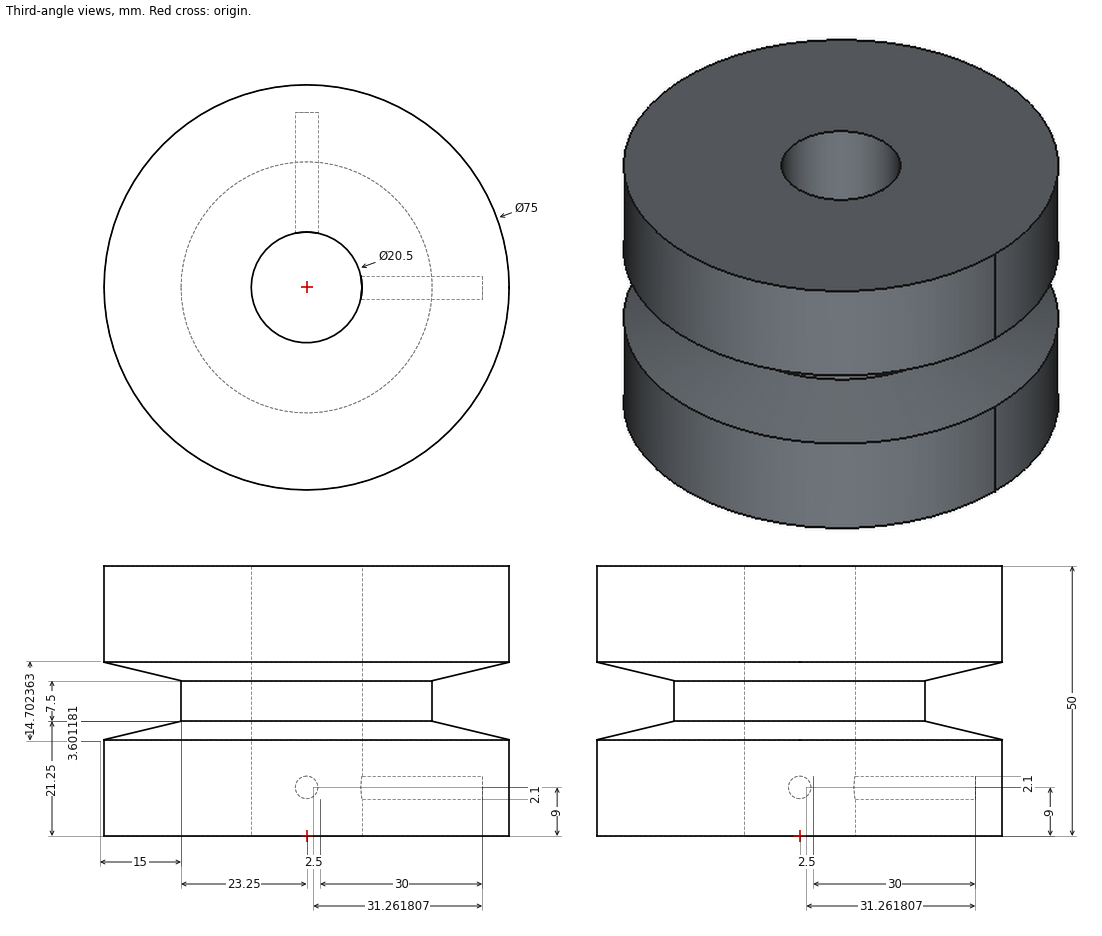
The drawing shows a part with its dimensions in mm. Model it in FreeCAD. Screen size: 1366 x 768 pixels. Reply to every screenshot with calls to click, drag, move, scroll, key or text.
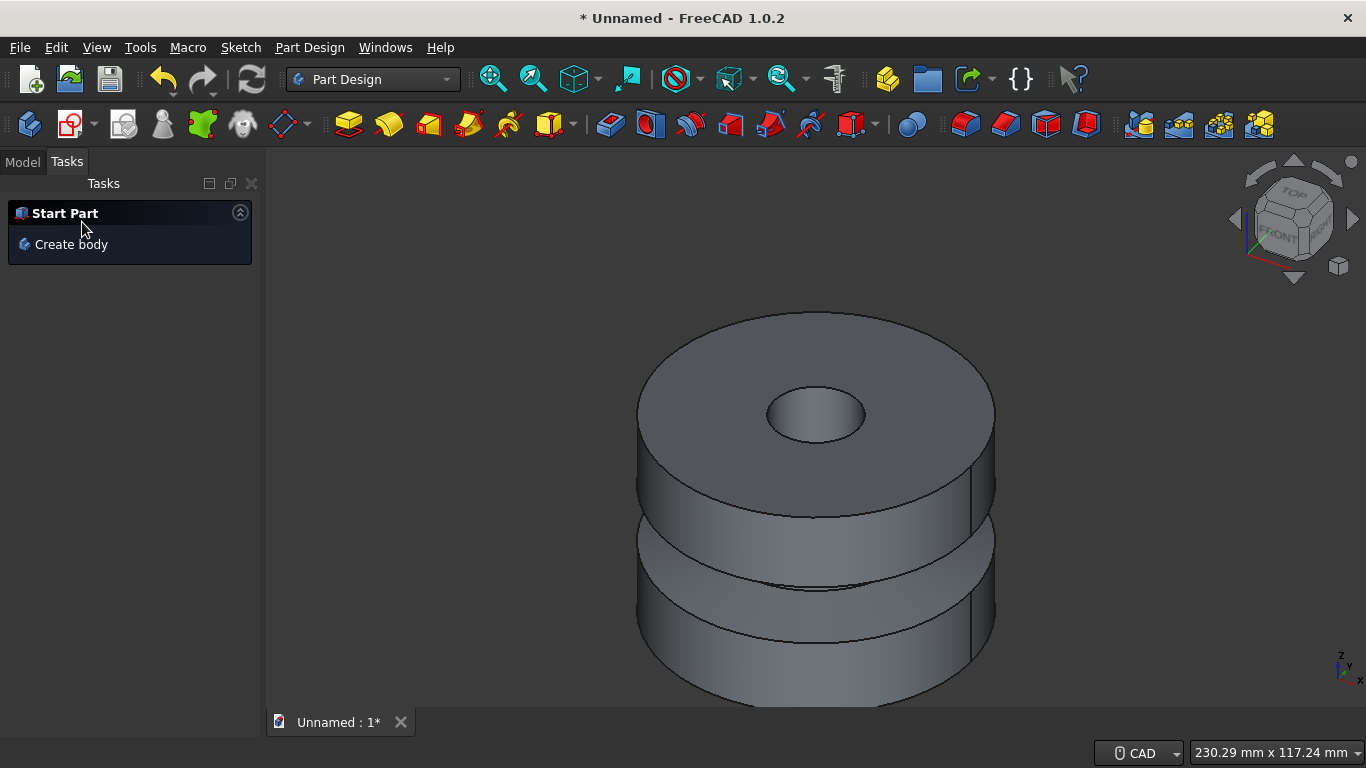
key(0)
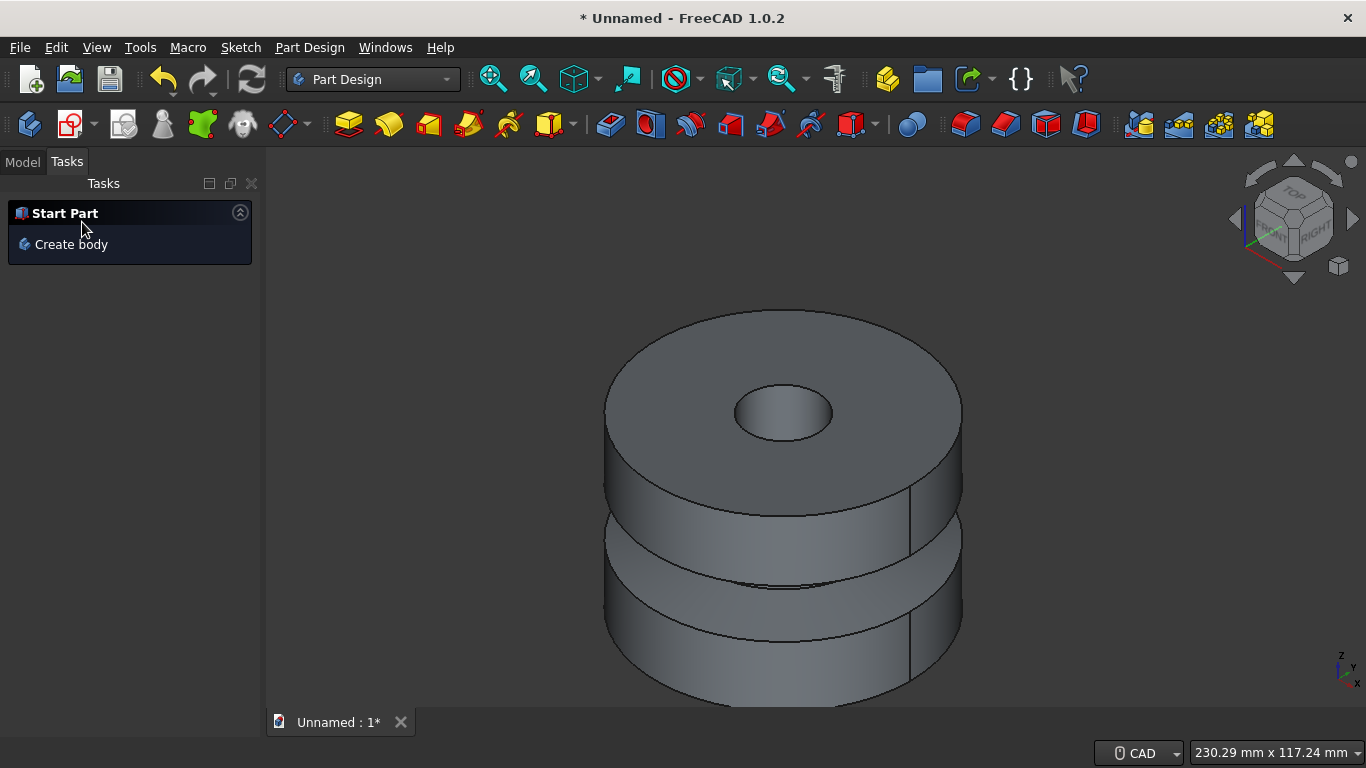
key(v)
key(f)